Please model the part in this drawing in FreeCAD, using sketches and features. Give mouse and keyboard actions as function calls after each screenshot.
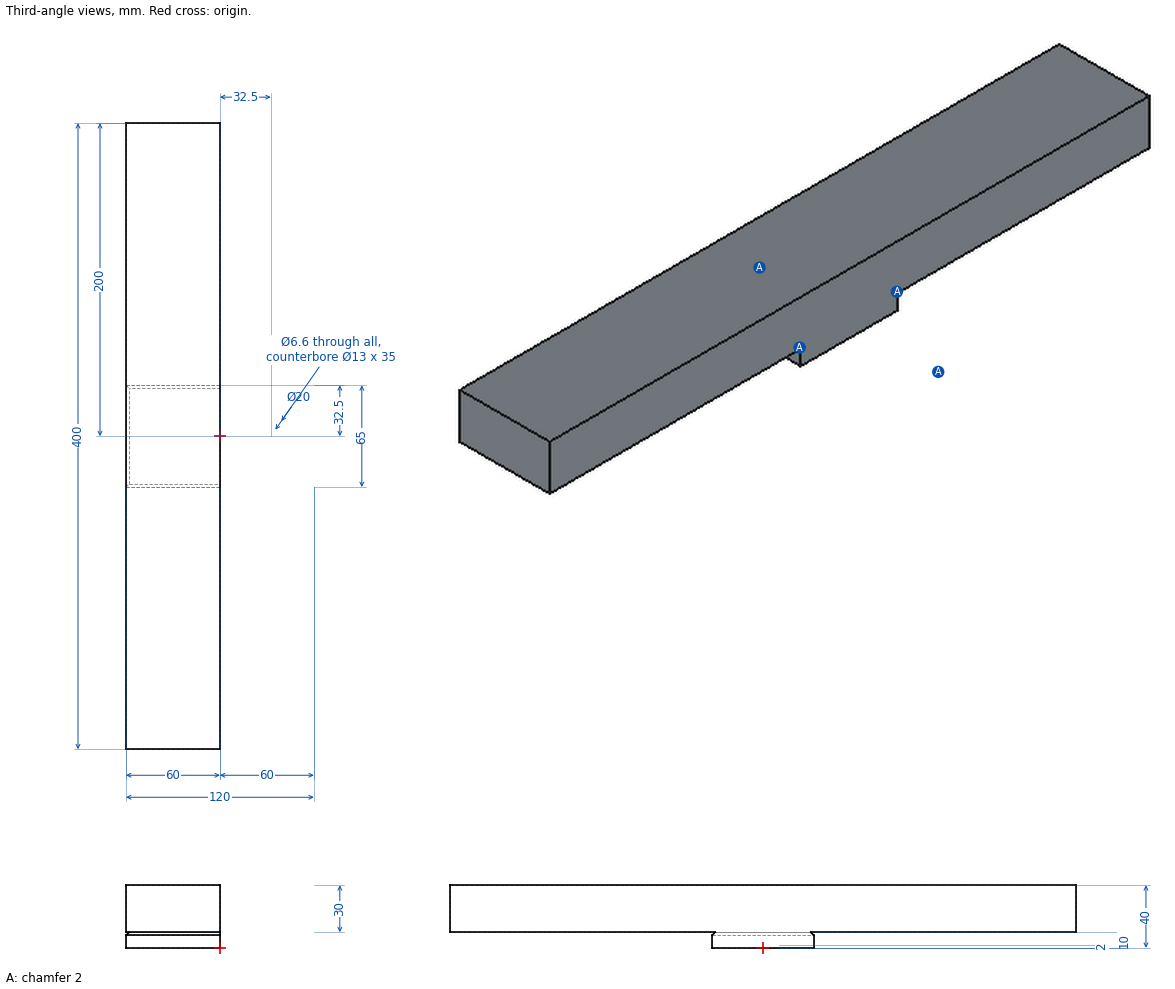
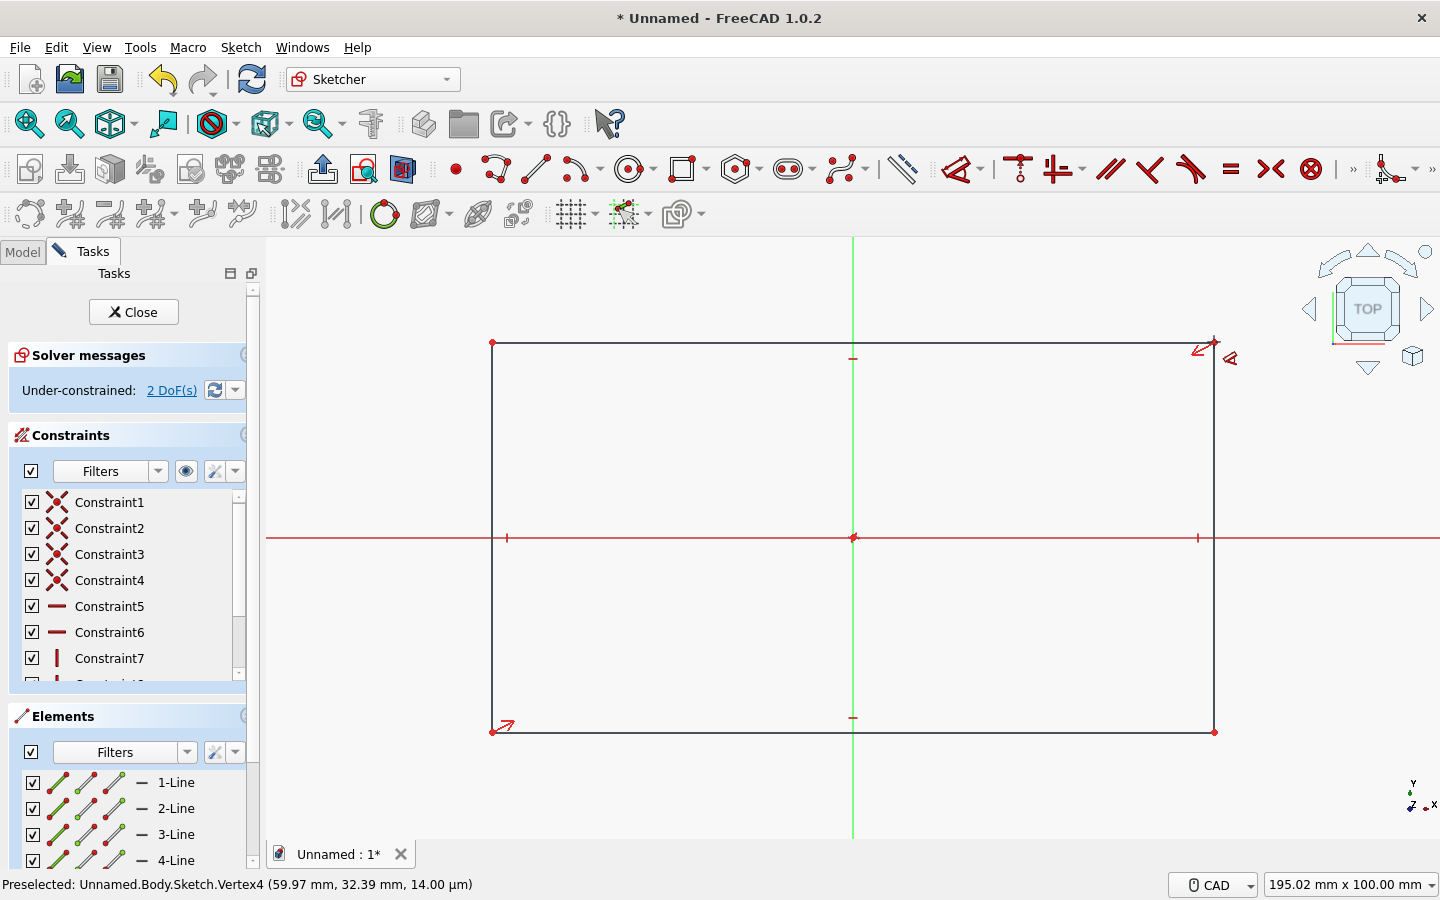
click(1214, 616)
click(1248, 448)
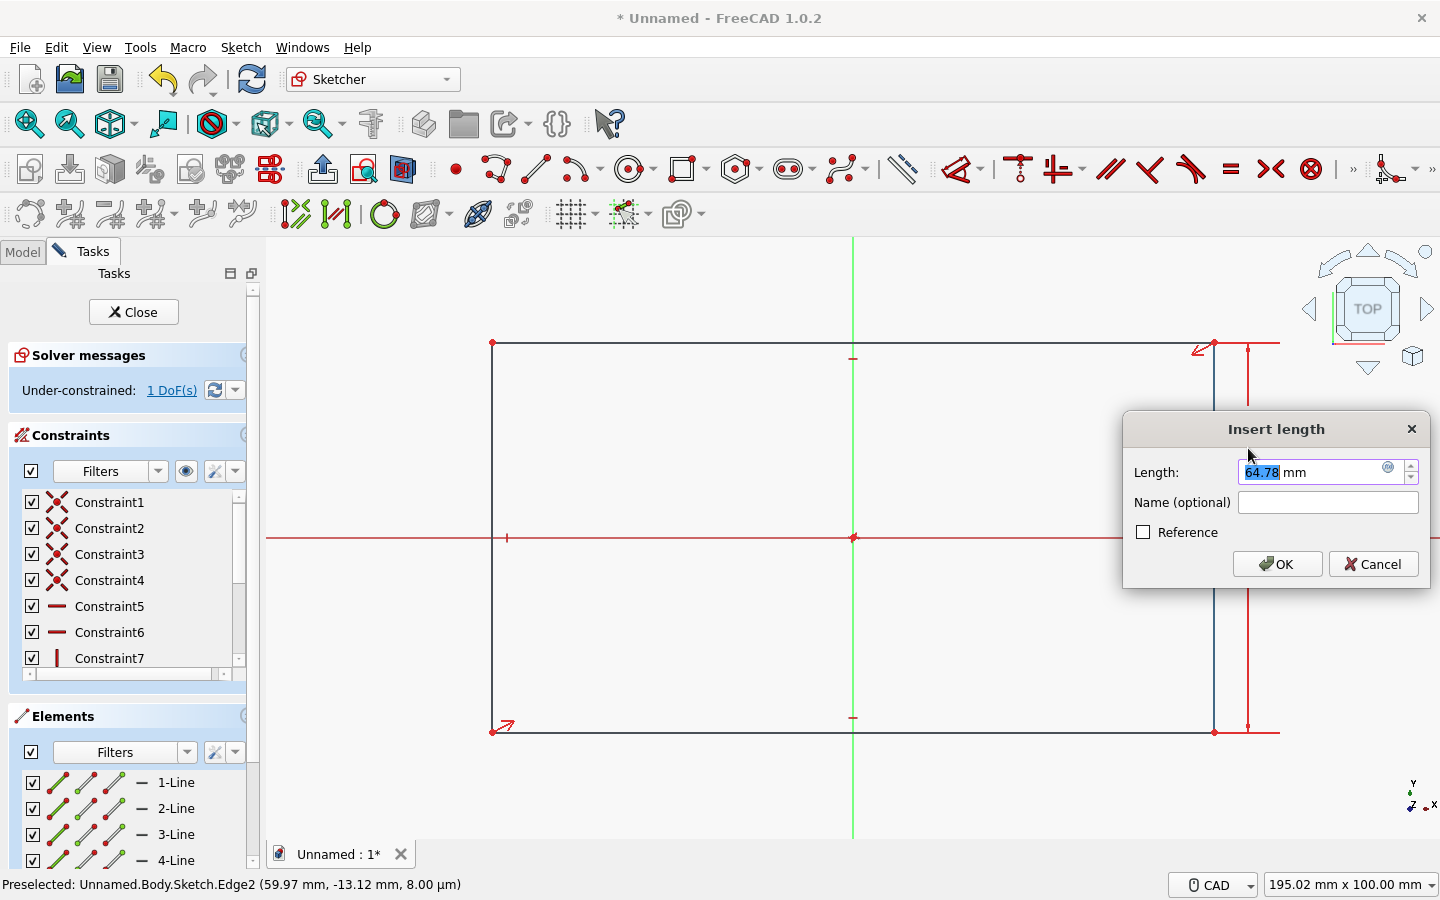
text(65)
key(Return)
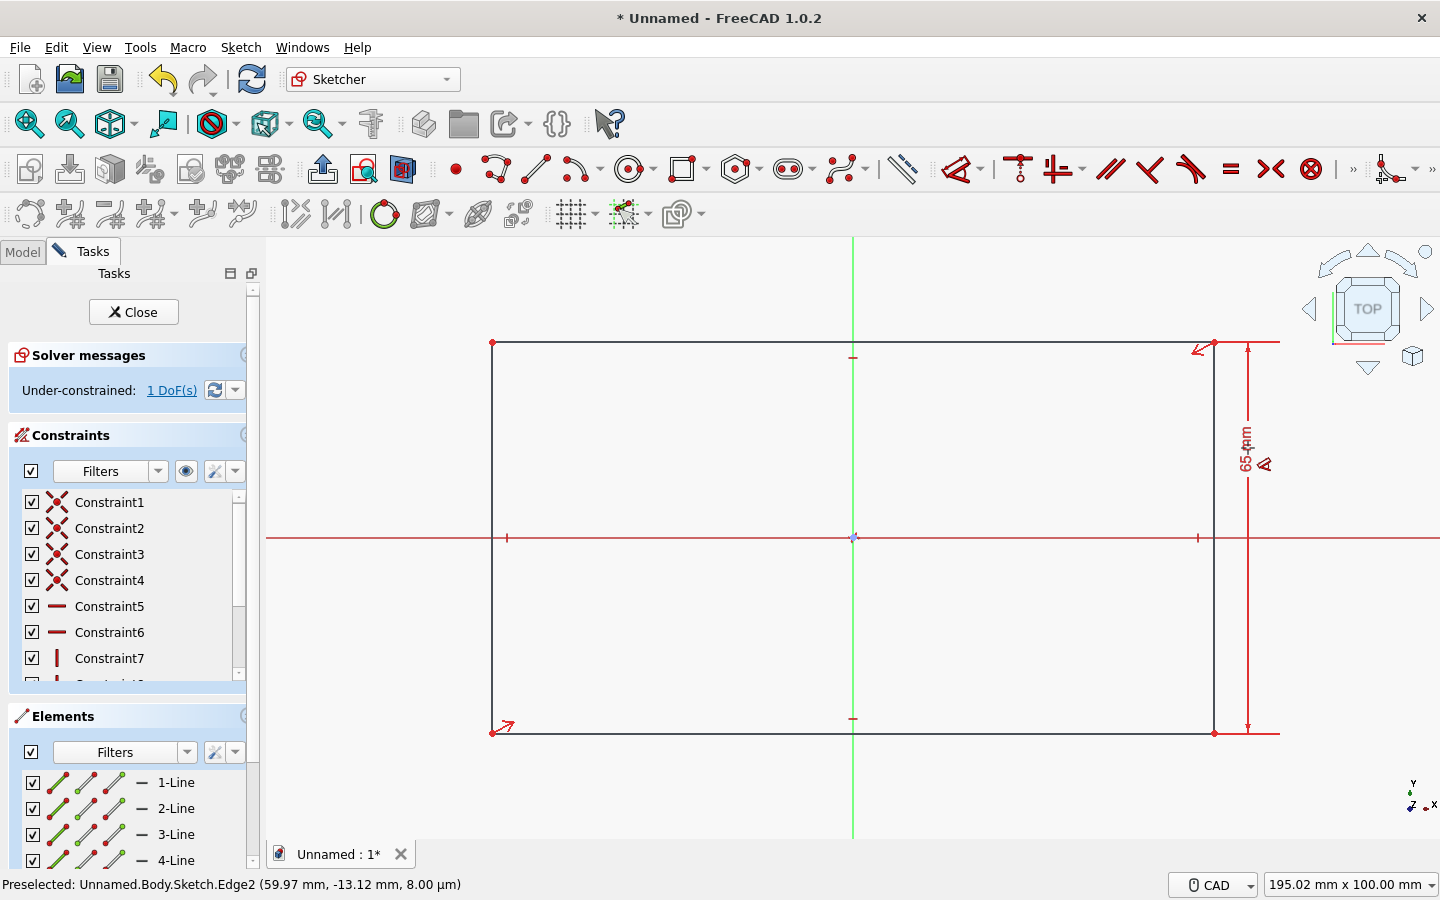
click(709, 734)
click(687, 768)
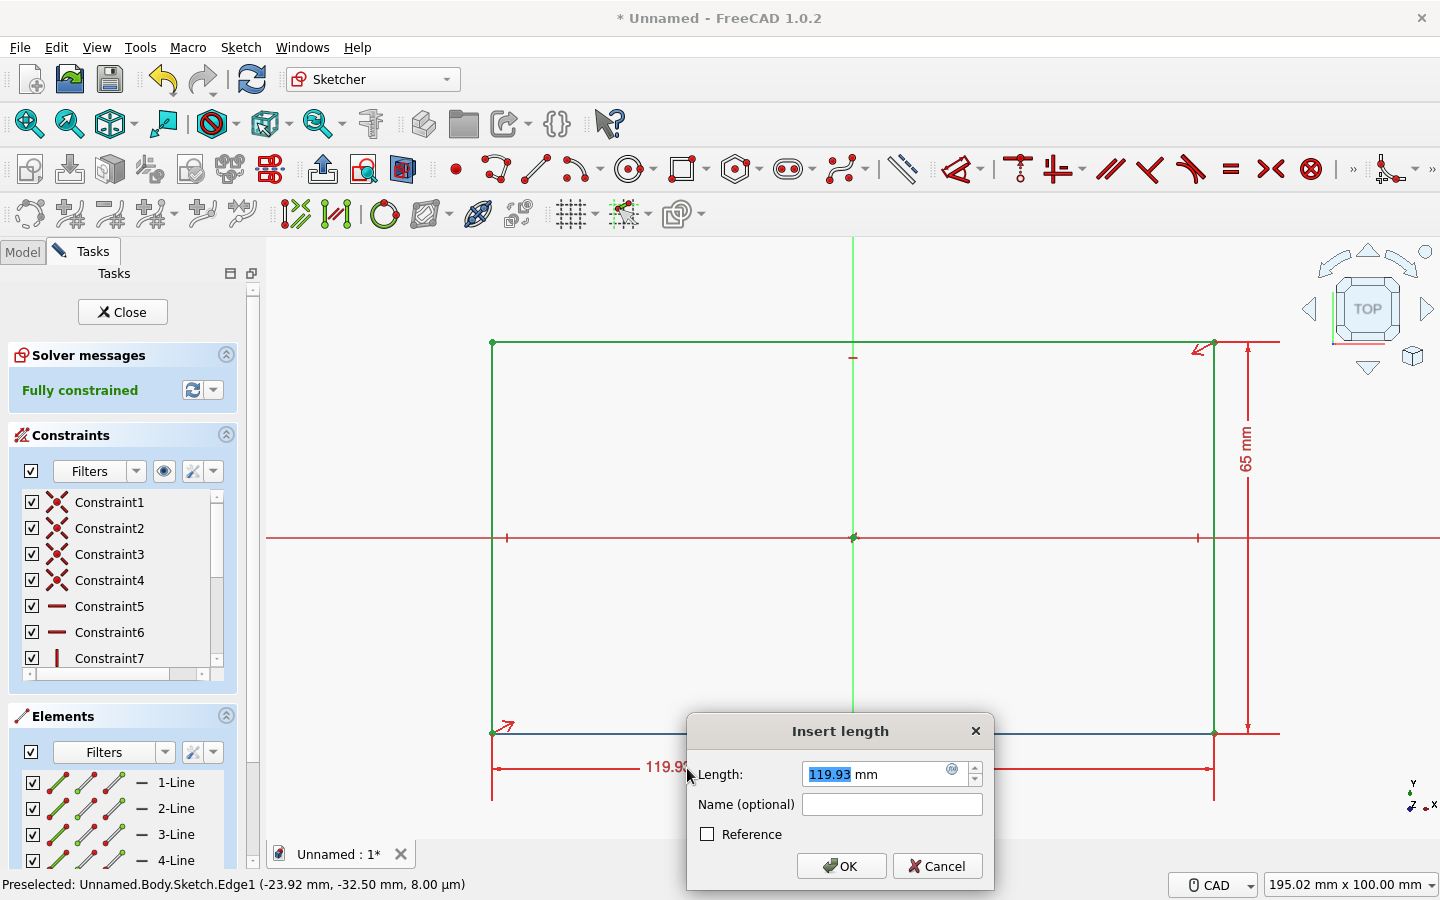
text(120)
key(Return)
key(Escape)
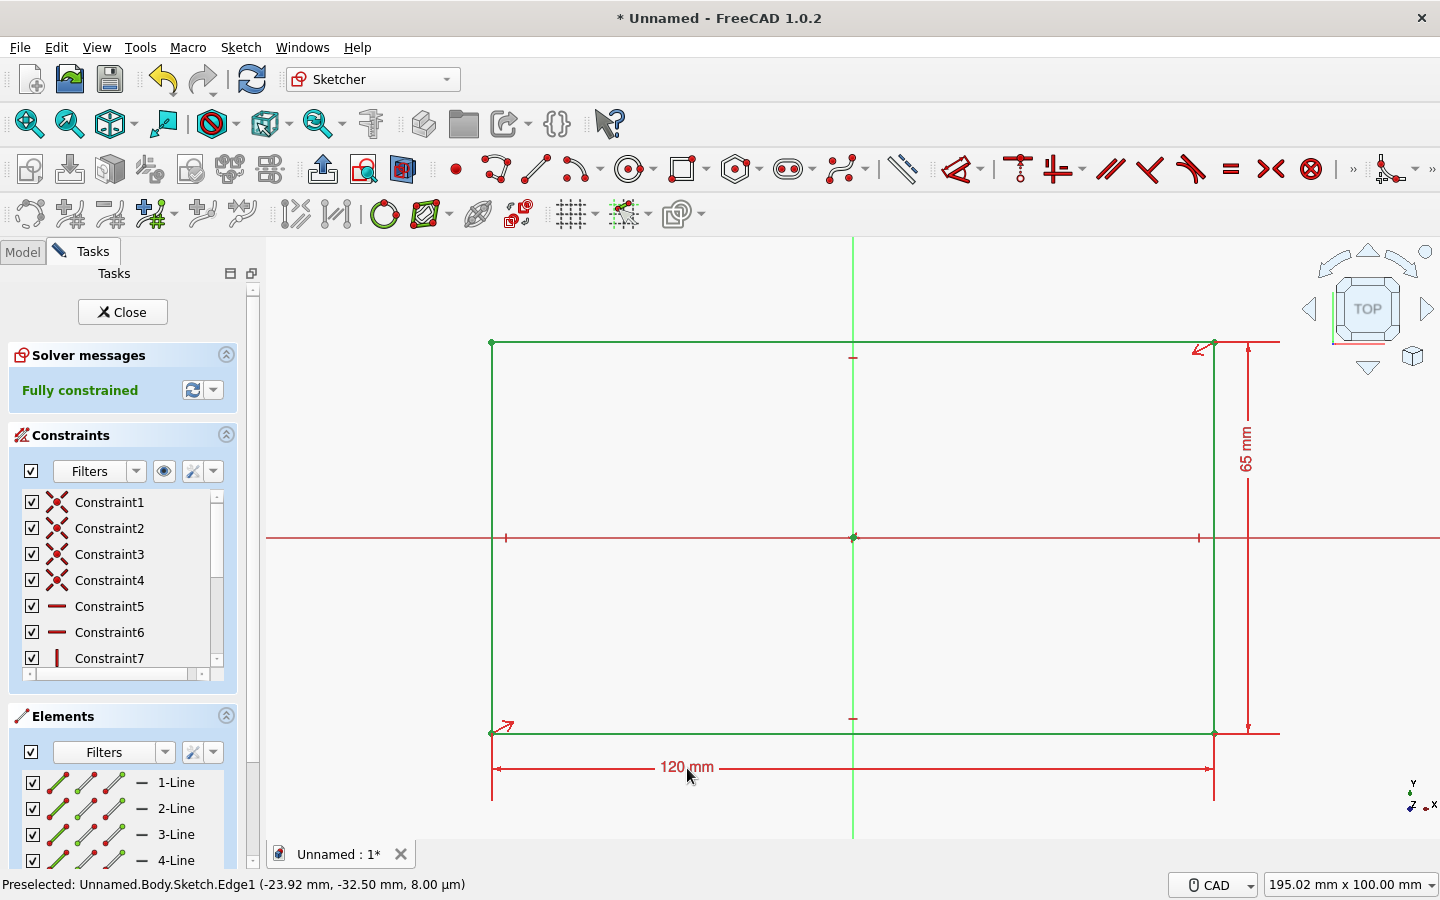
click(123, 312)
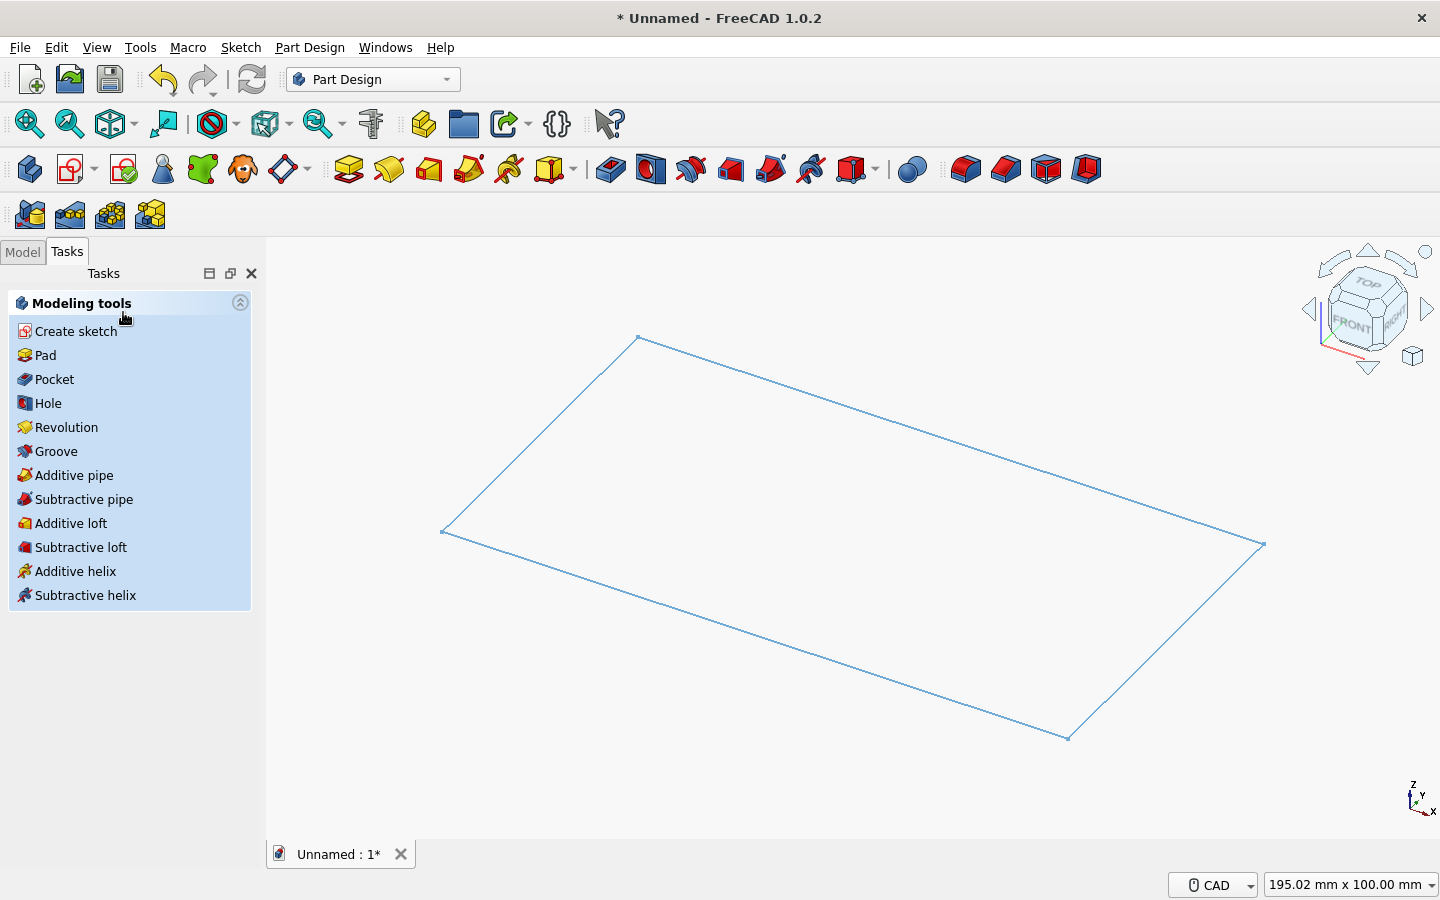
click(350, 170)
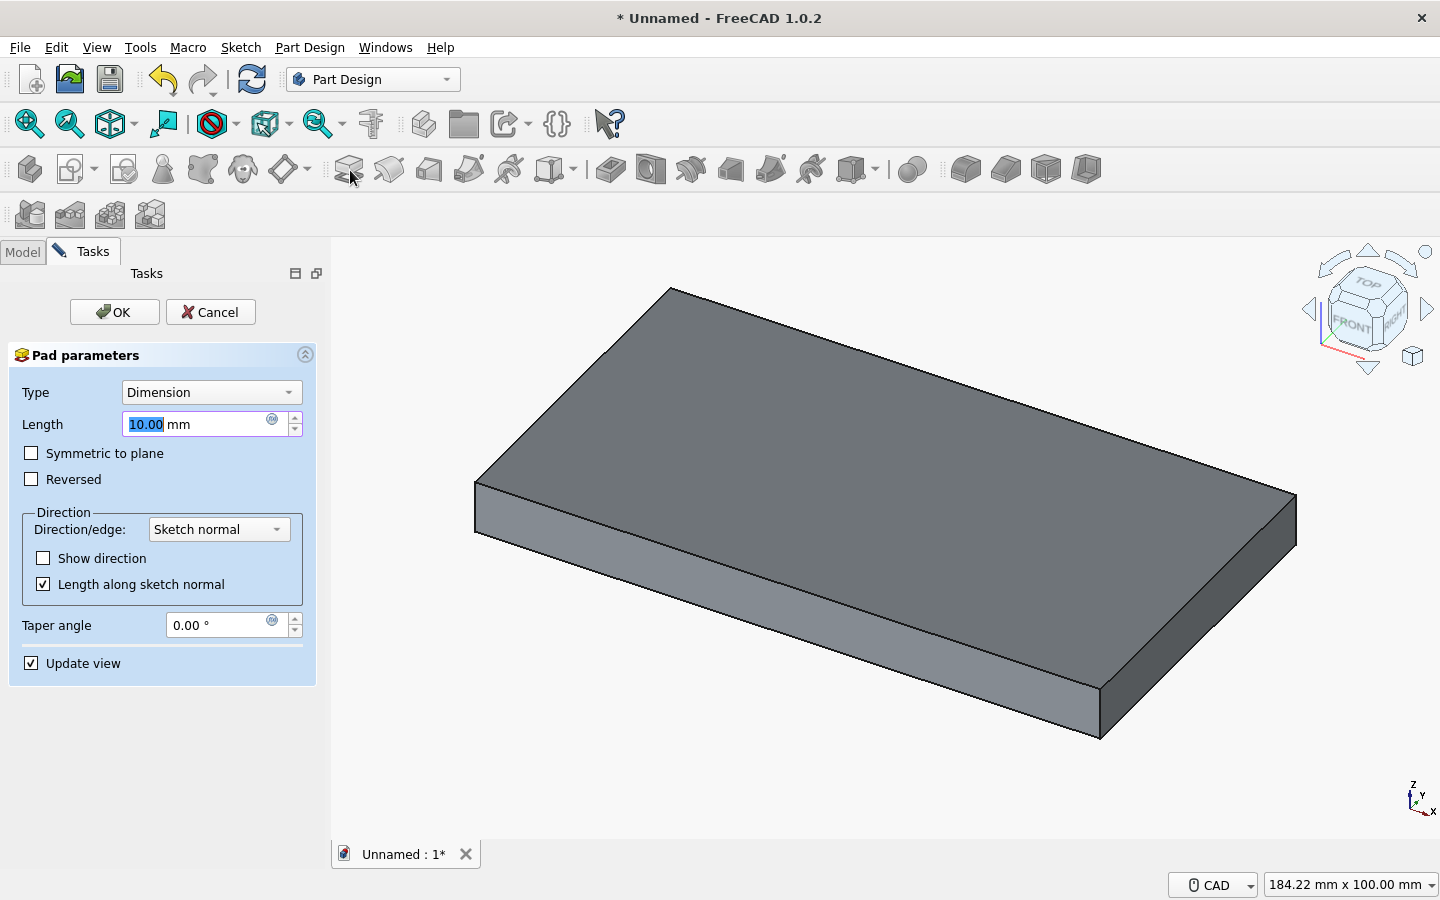
text(10)
key(Tab)